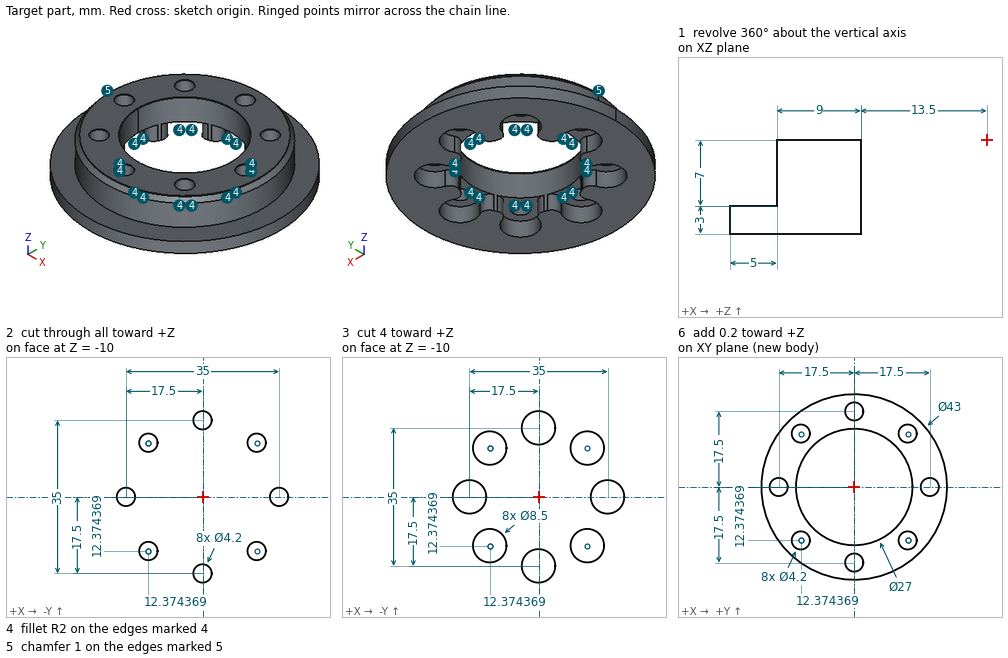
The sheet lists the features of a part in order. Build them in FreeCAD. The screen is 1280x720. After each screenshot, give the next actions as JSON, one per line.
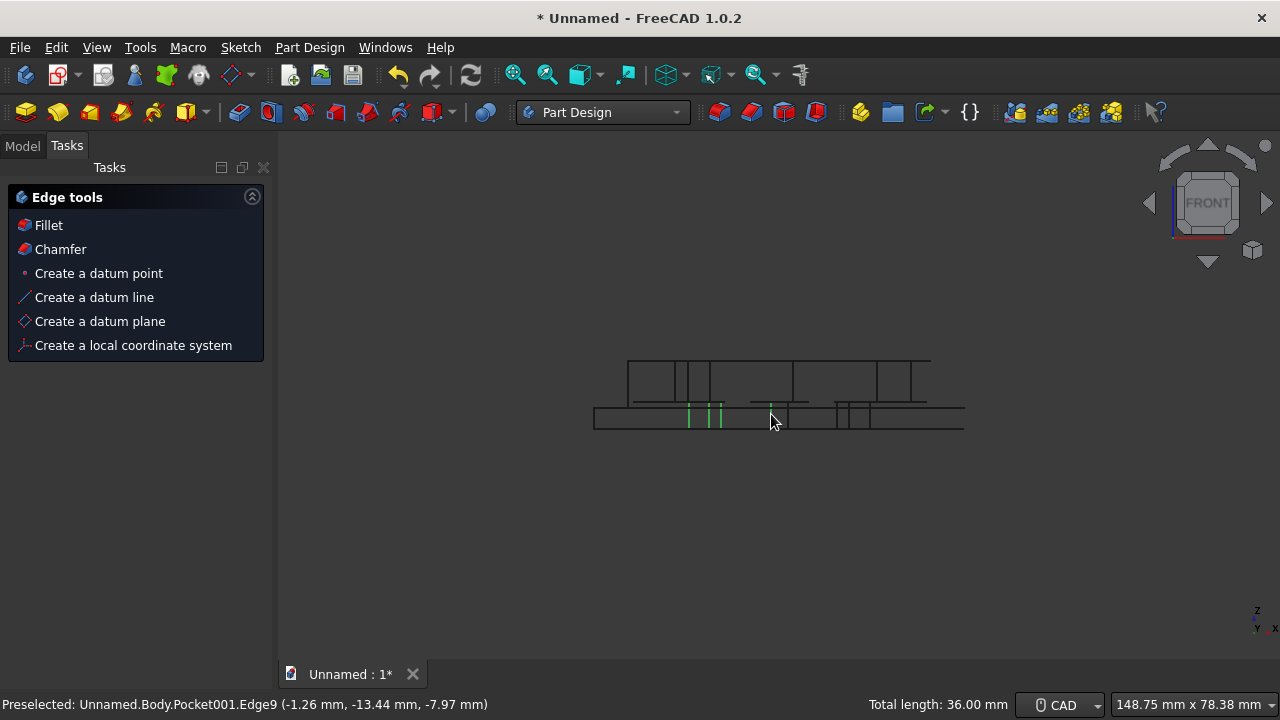
{"action": "left_click", "coordinate": [788, 414], "text": "ctrl"}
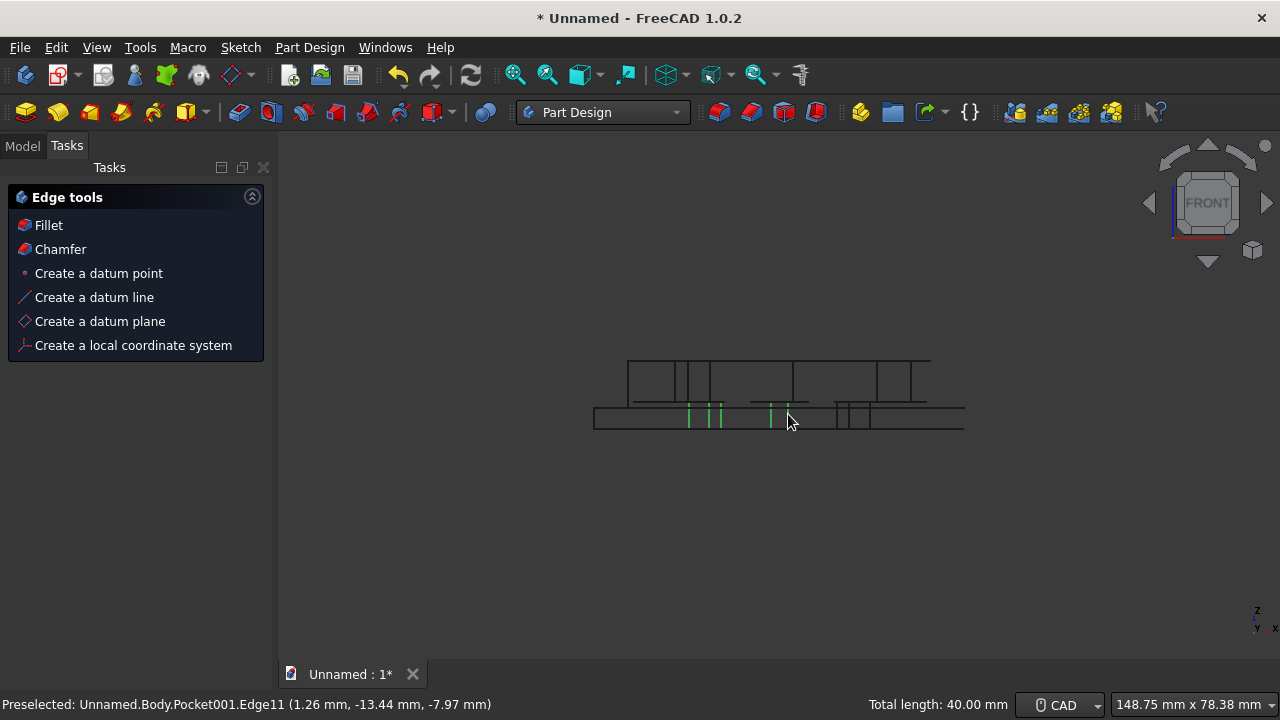
{"action": "left_click", "coordinate": [837, 414], "text": "ctrl"}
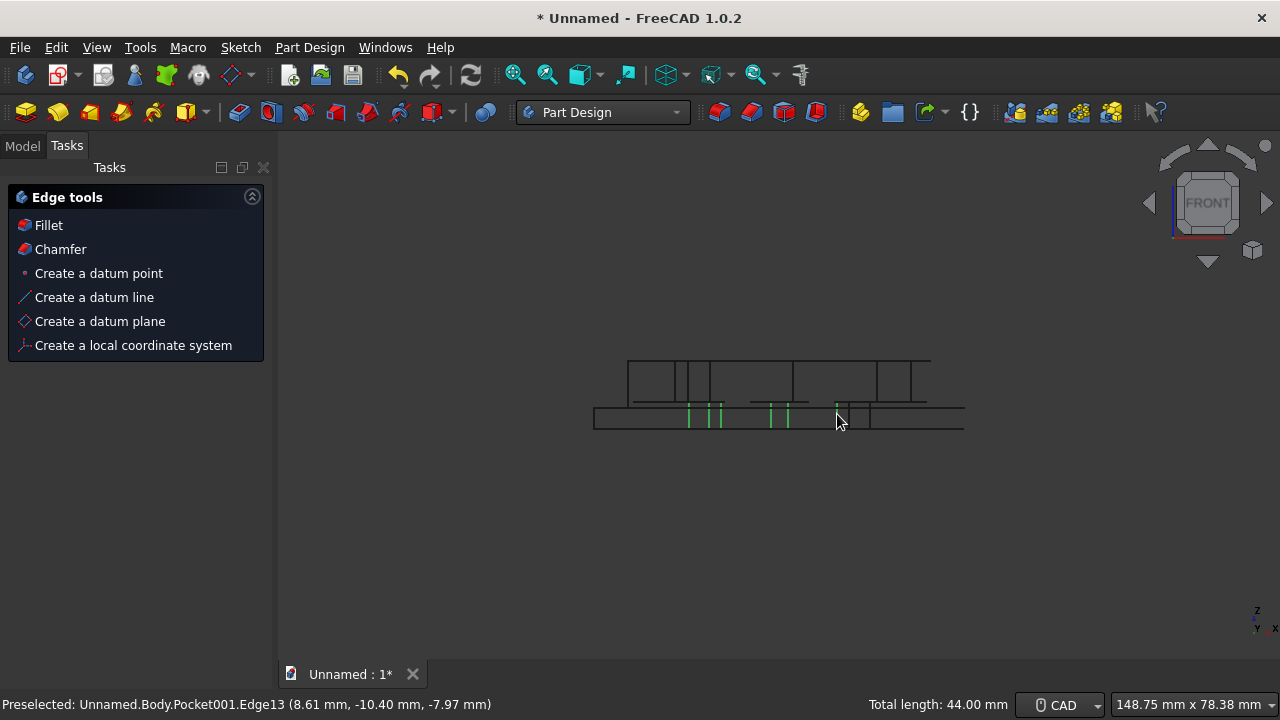
{"action": "left_click", "coordinate": [849, 414], "text": "ctrl"}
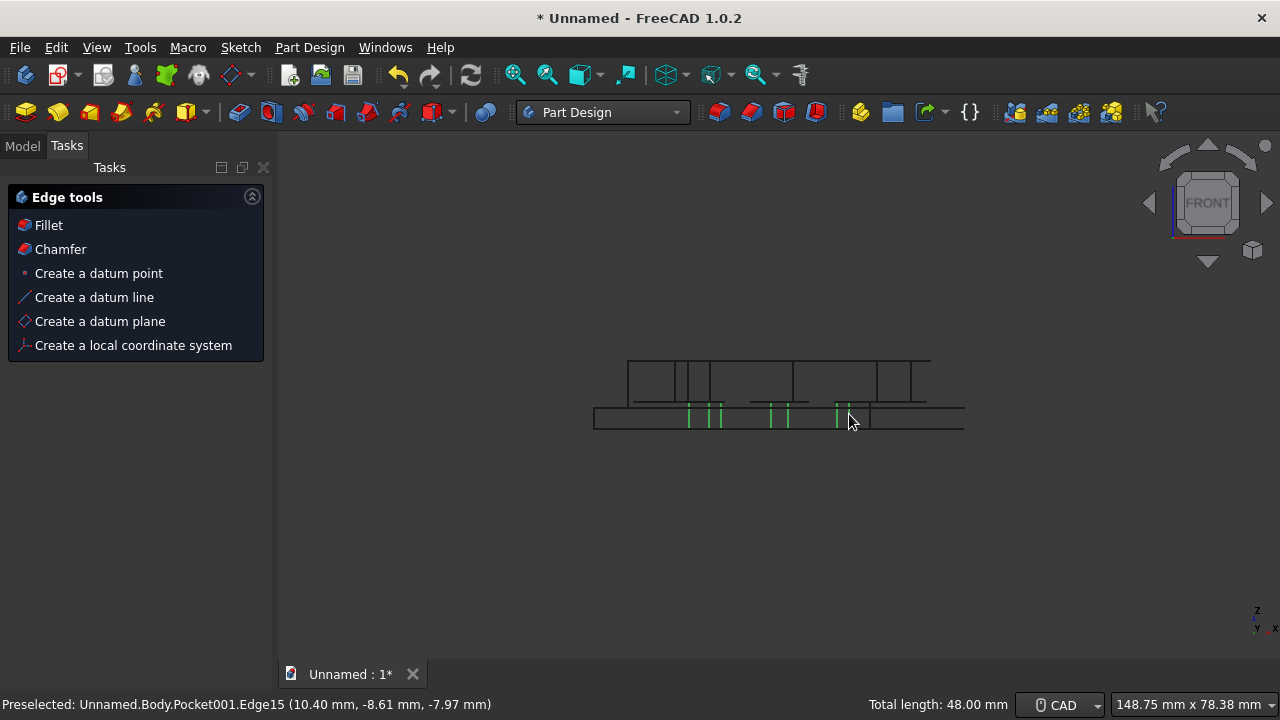
{"action": "left_click", "coordinate": [870, 414], "text": "ctrl"}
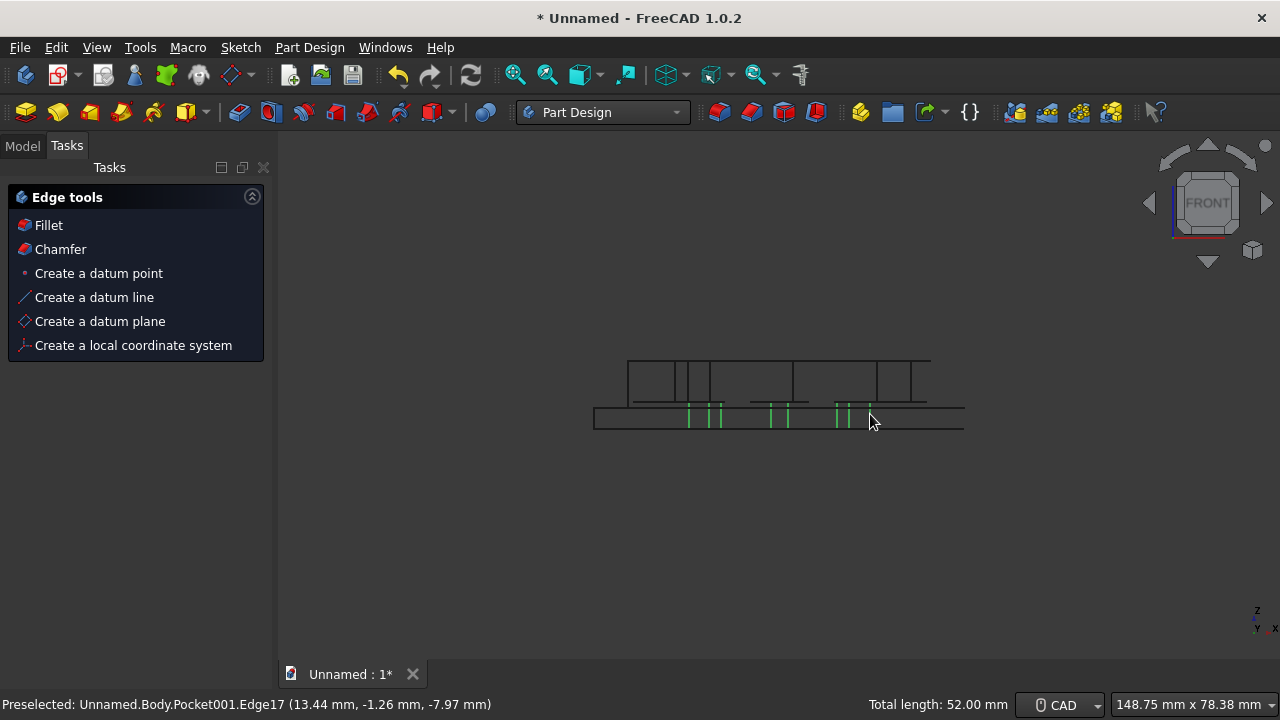
{"action": "key", "text": "3"}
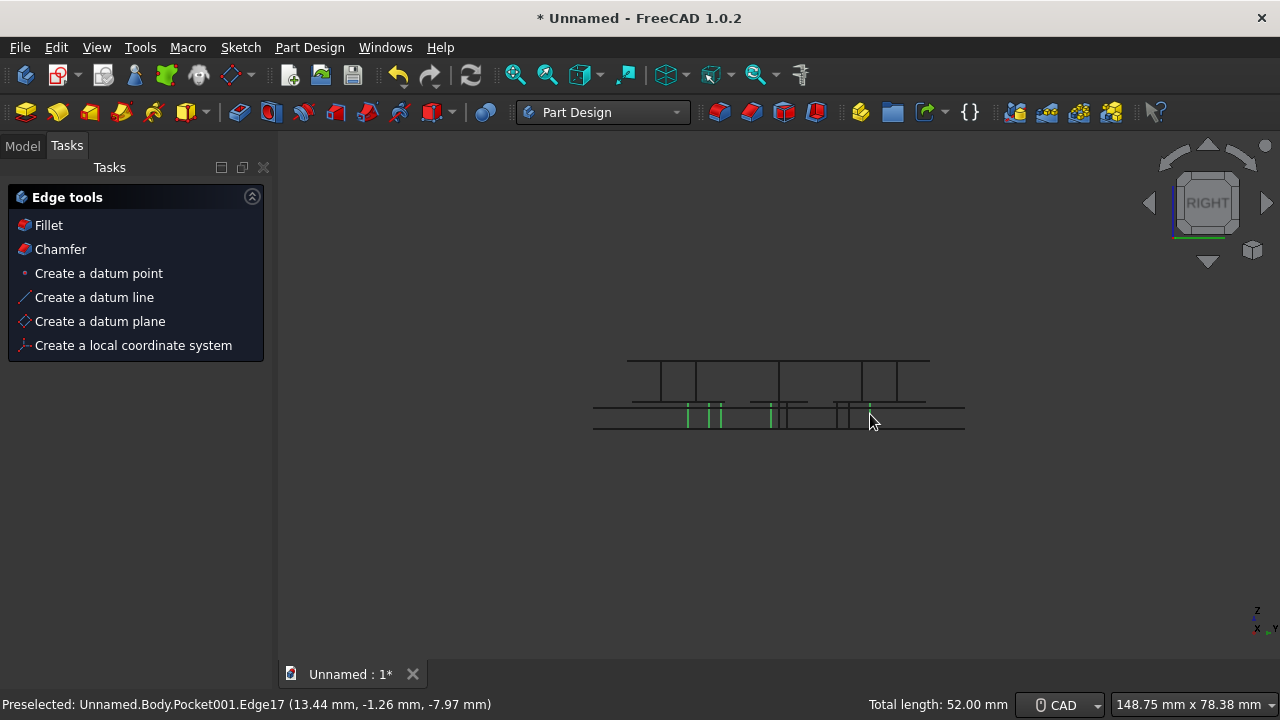
{"action": "key", "text": "v f"}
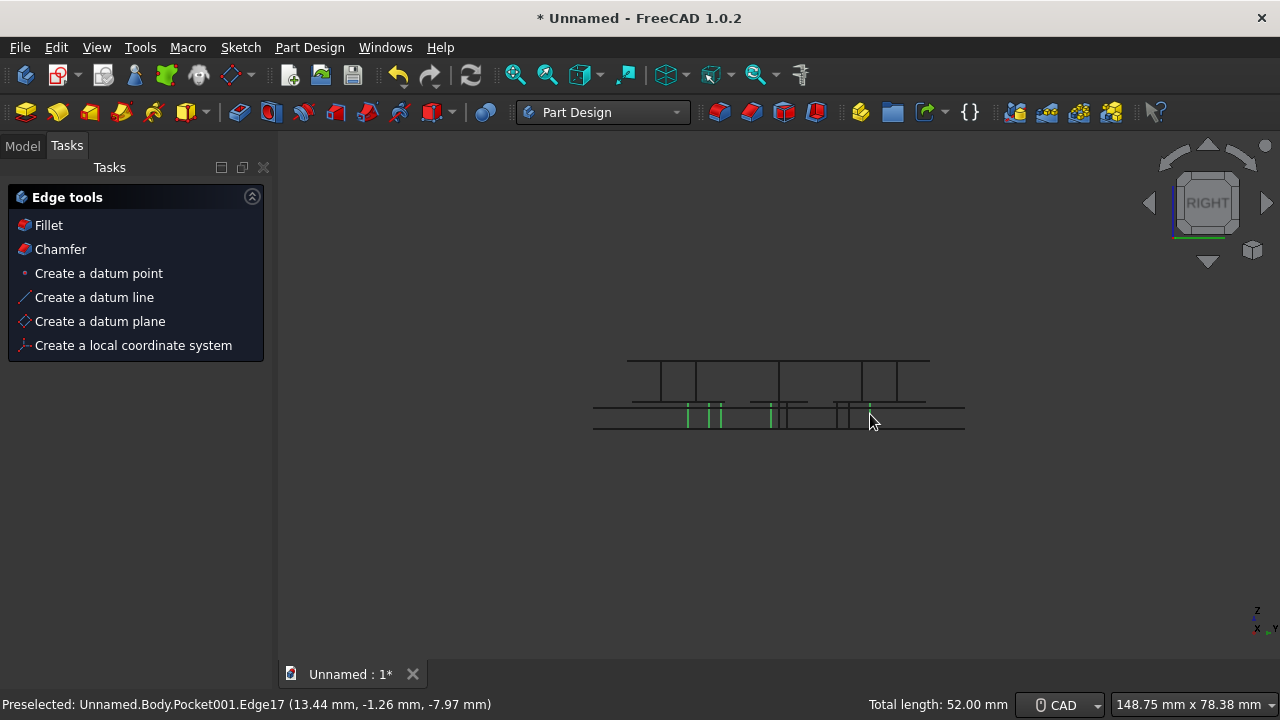
{"action": "left_click", "coordinate": [787, 414], "text": "ctrl"}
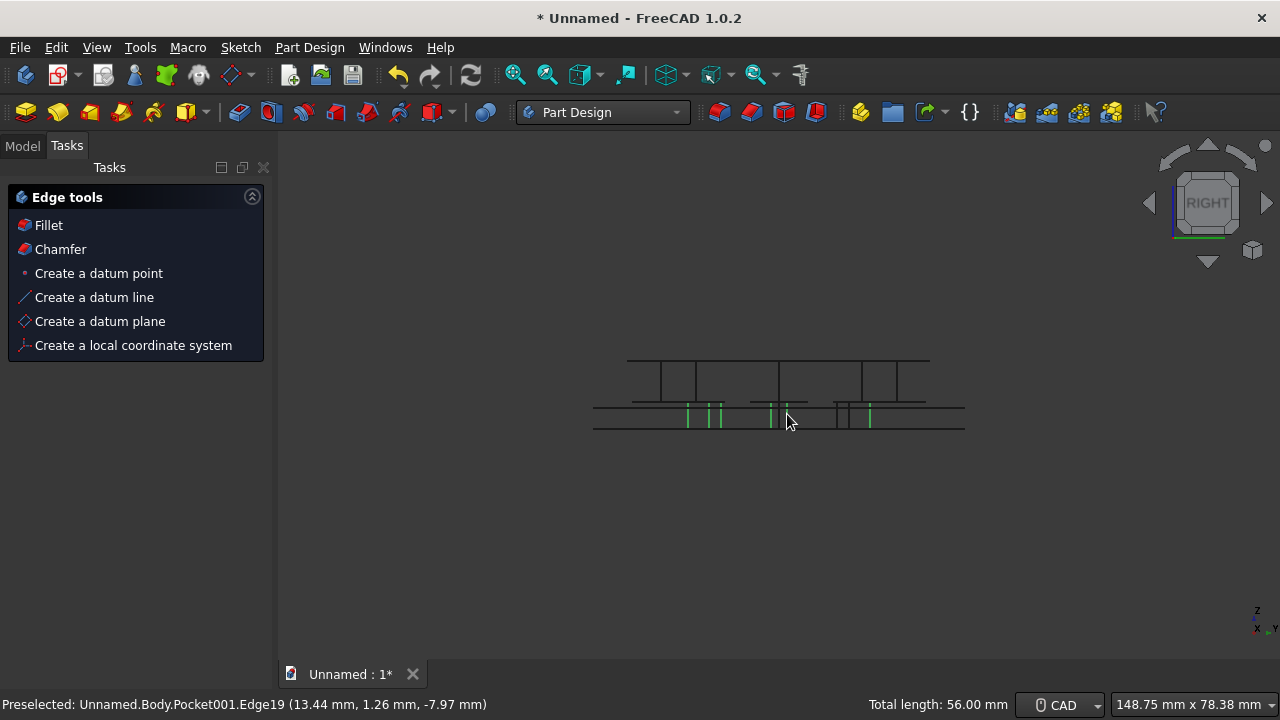
{"action": "left_click", "coordinate": [837, 414], "text": "ctrl"}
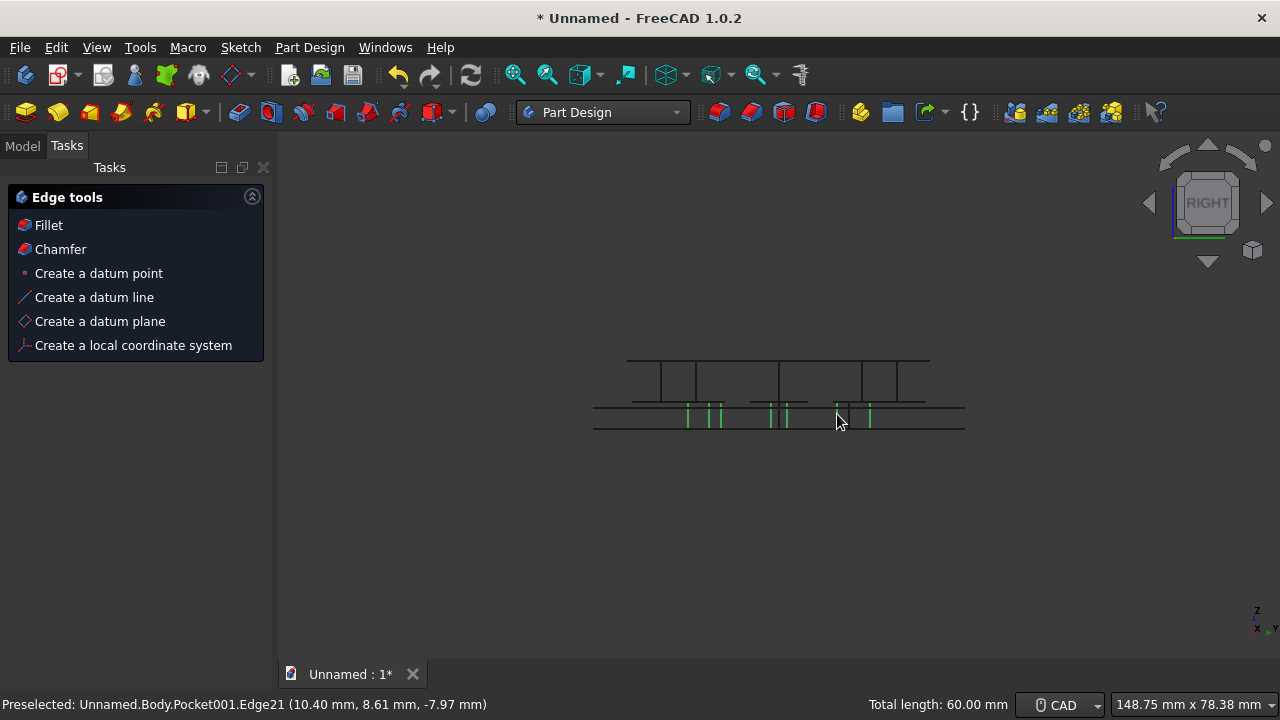
{"action": "left_click", "coordinate": [849, 414], "text": "ctrl"}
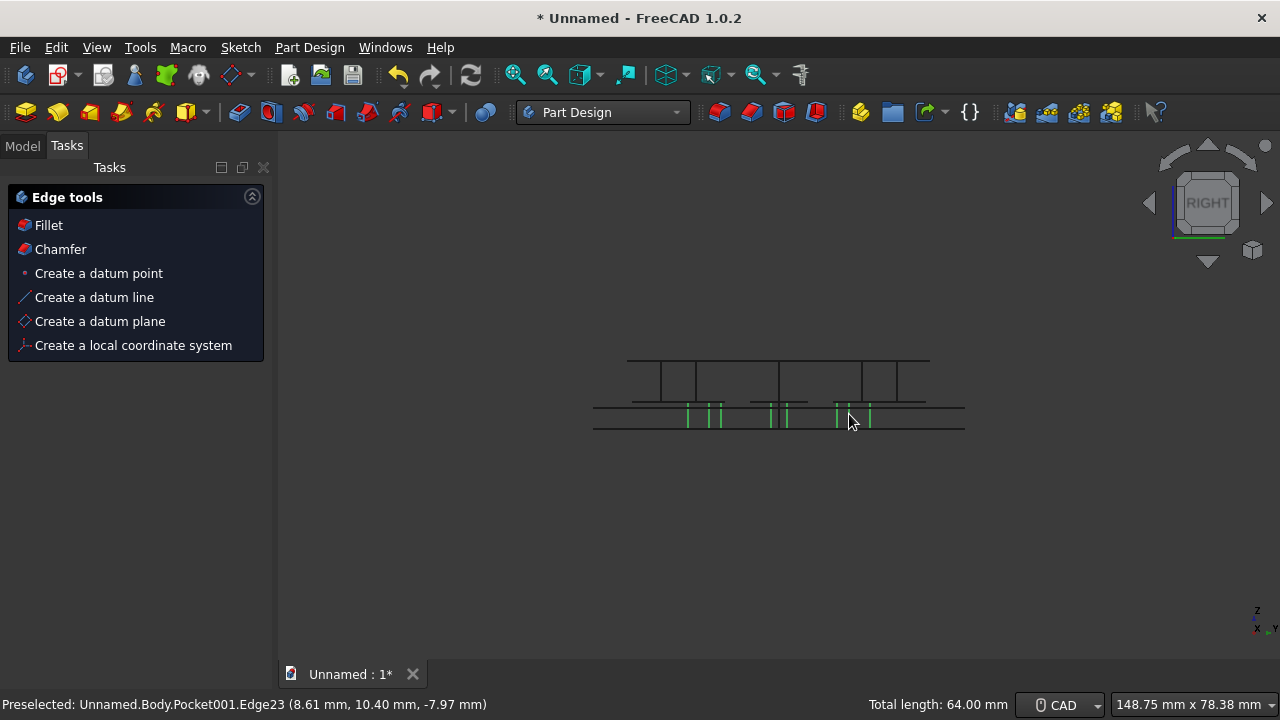
{"action": "key", "text": "v 1"}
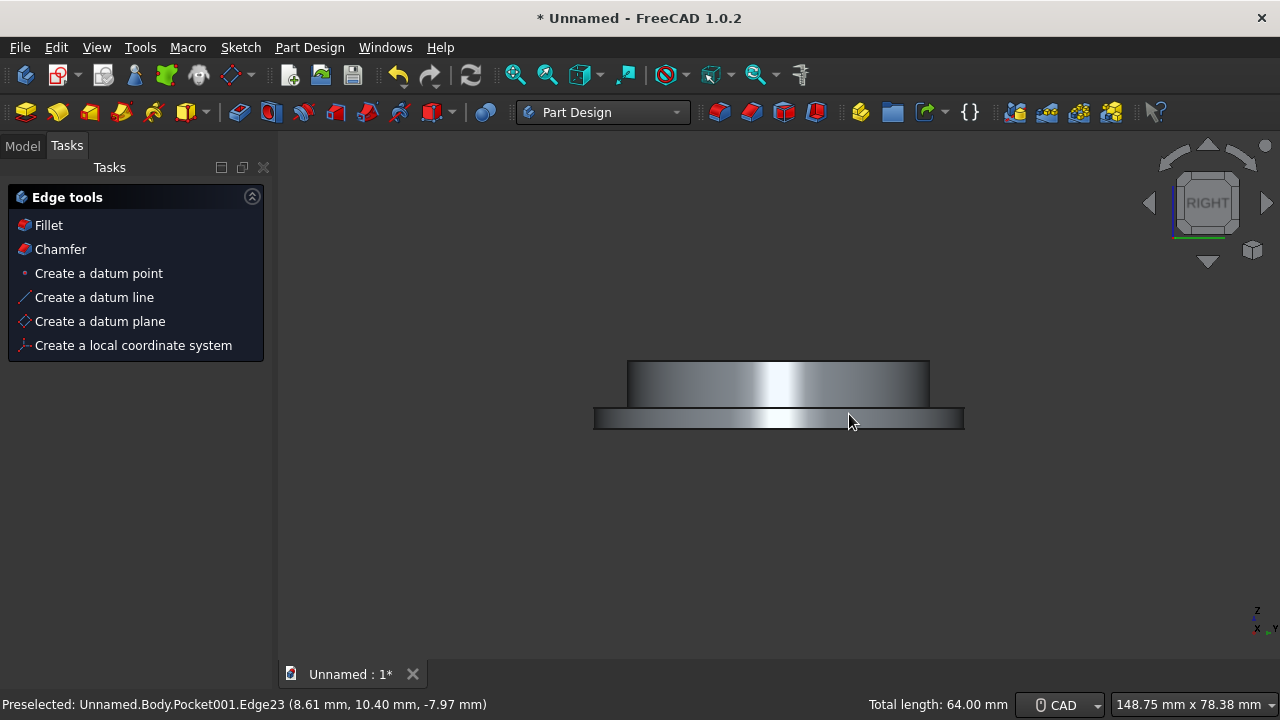
{"action": "left_click", "coordinate": [720, 112]}